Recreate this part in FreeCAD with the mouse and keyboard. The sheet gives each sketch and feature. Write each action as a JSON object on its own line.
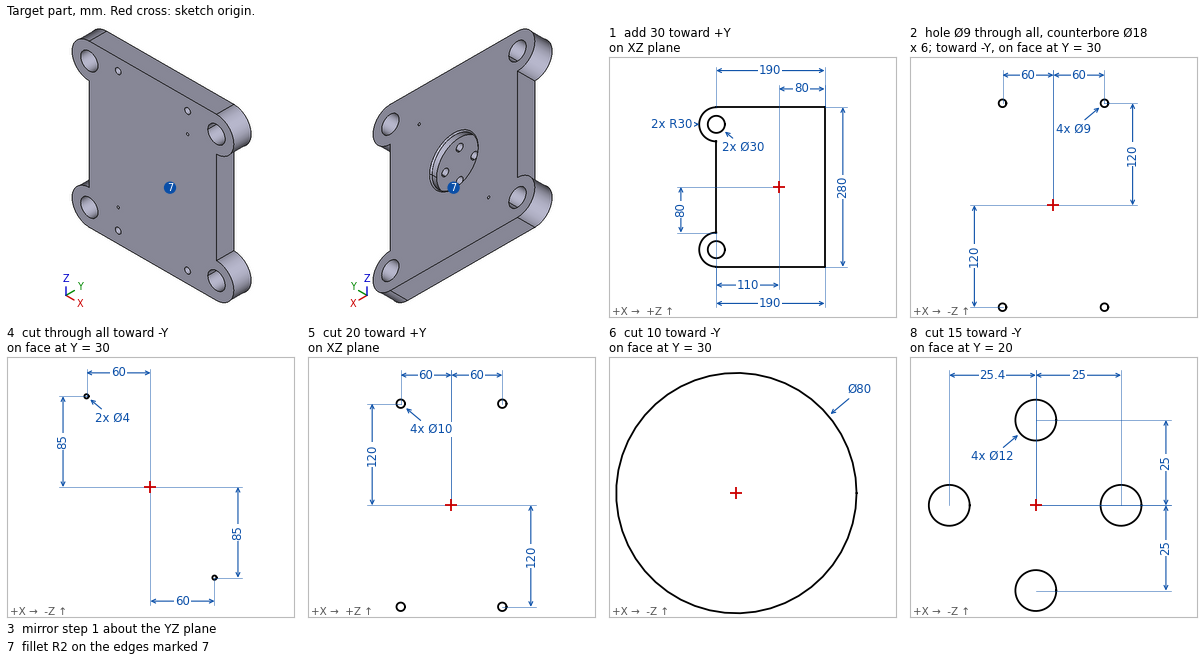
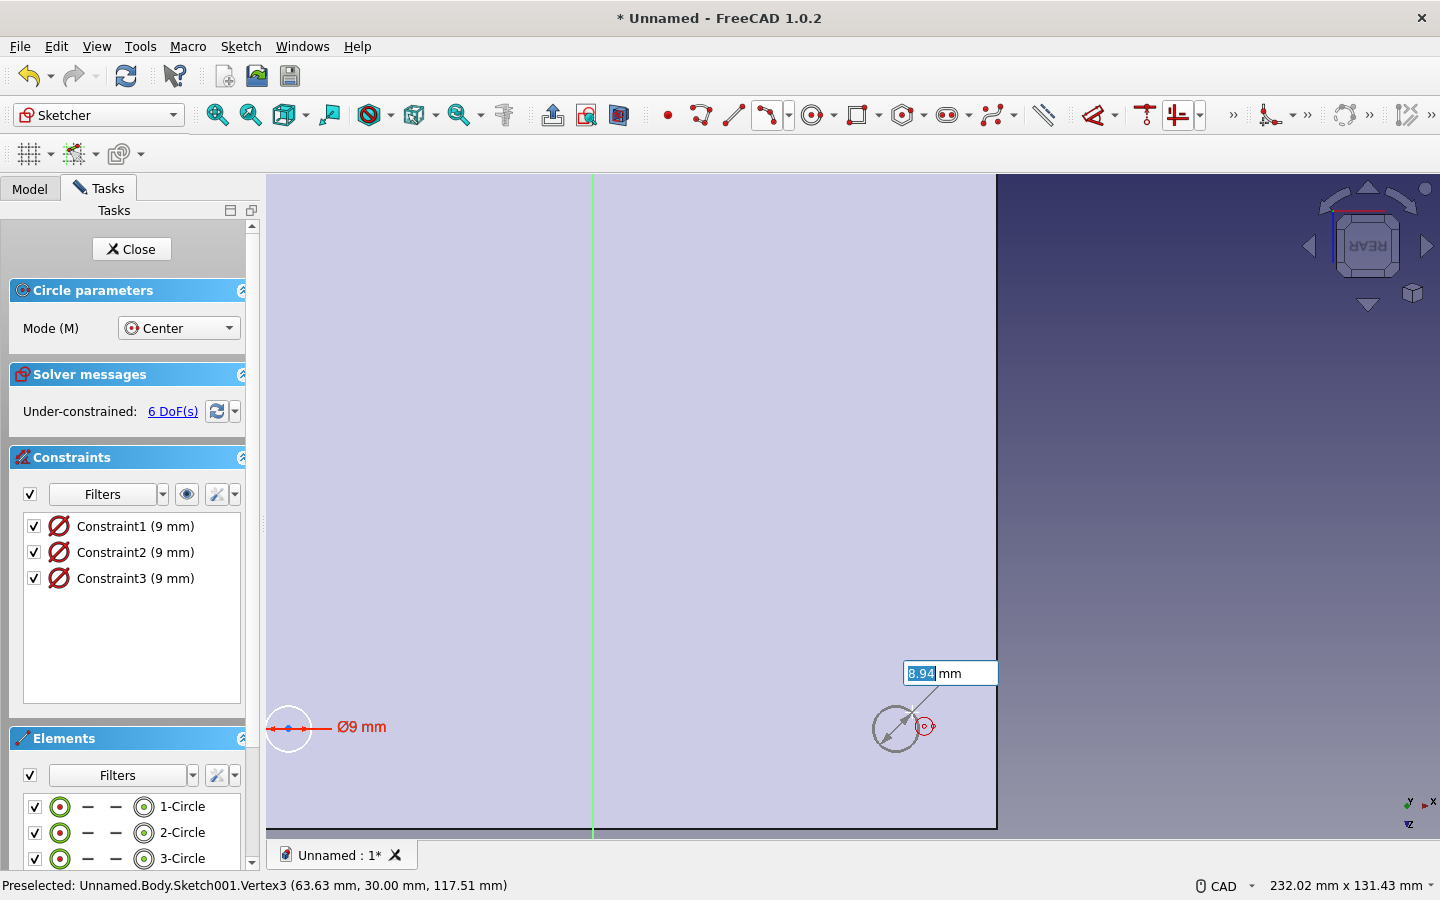
{"action": "type", "text": "9"}
{"action": "key", "text": "Return"}
{"action": "key", "text": "Escape"}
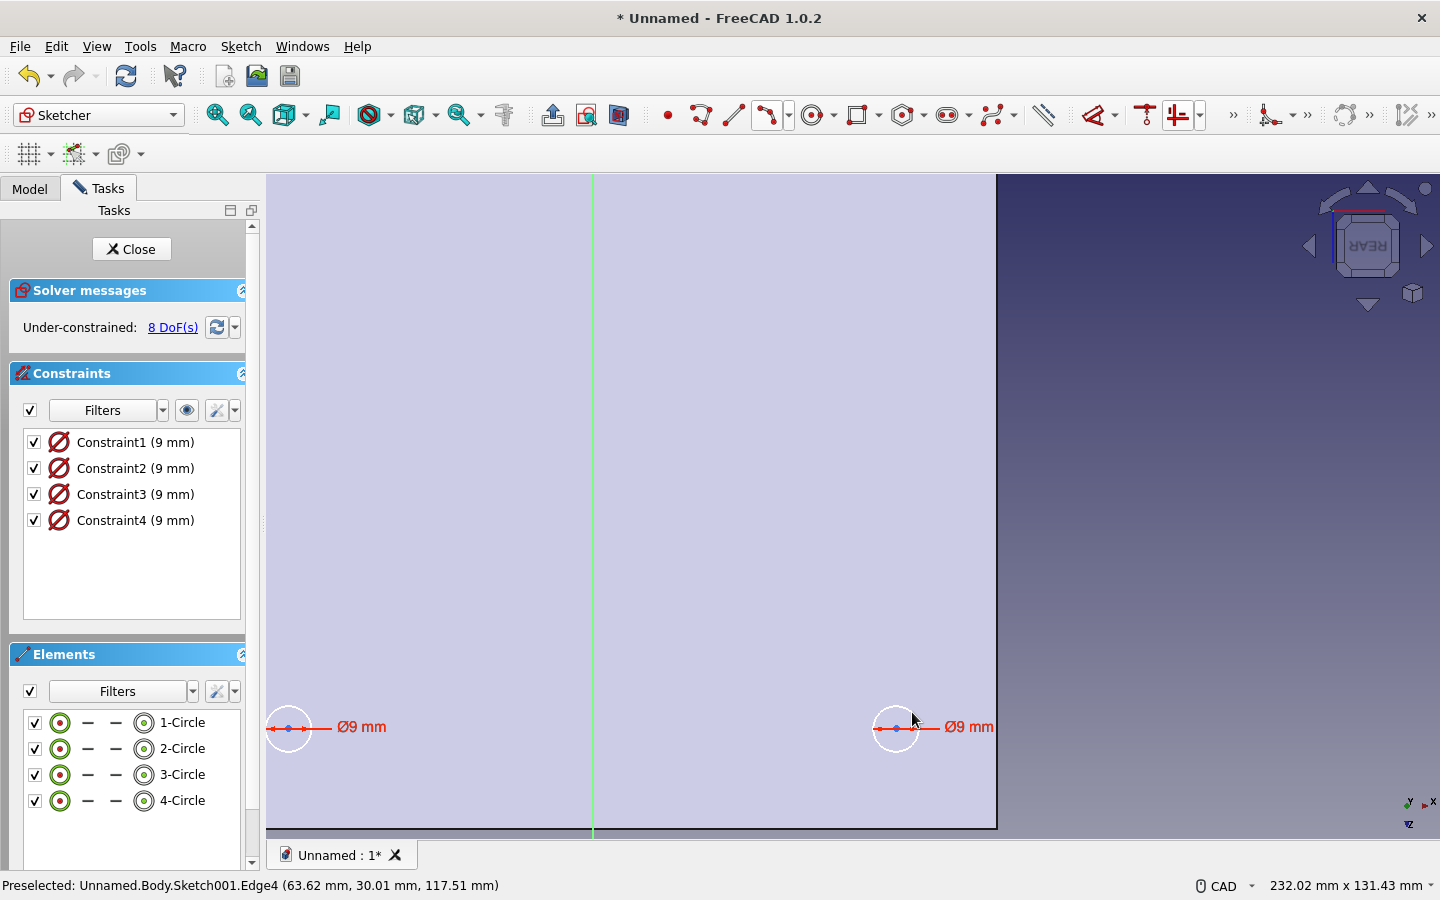
{"action": "scroll", "coordinate": [896, 731], "scroll_direction": "down", "scroll_amount": 5}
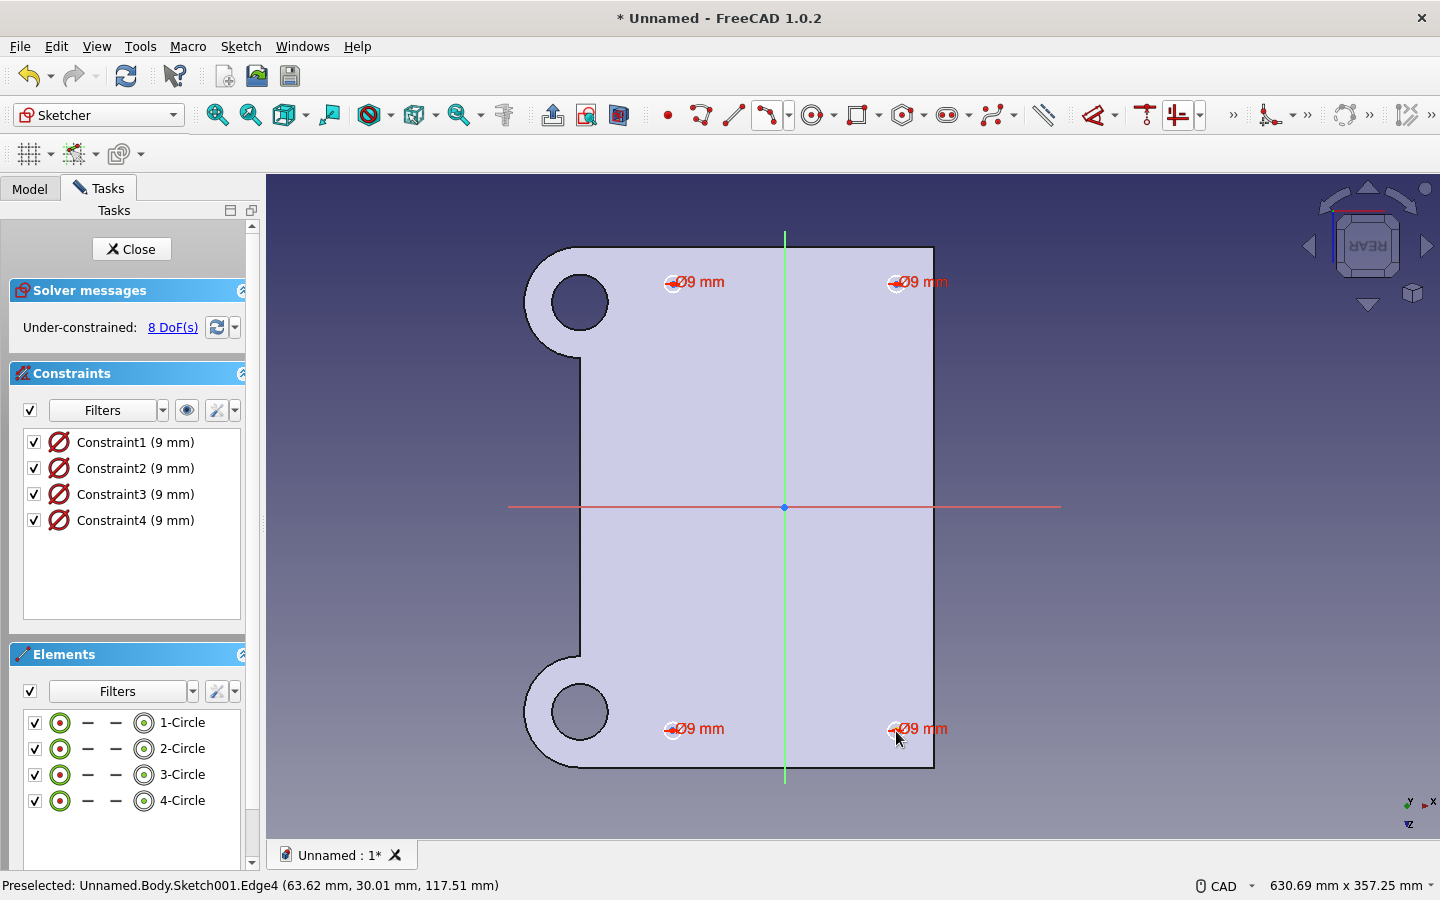
{"action": "left_click", "coordinate": [896, 284]}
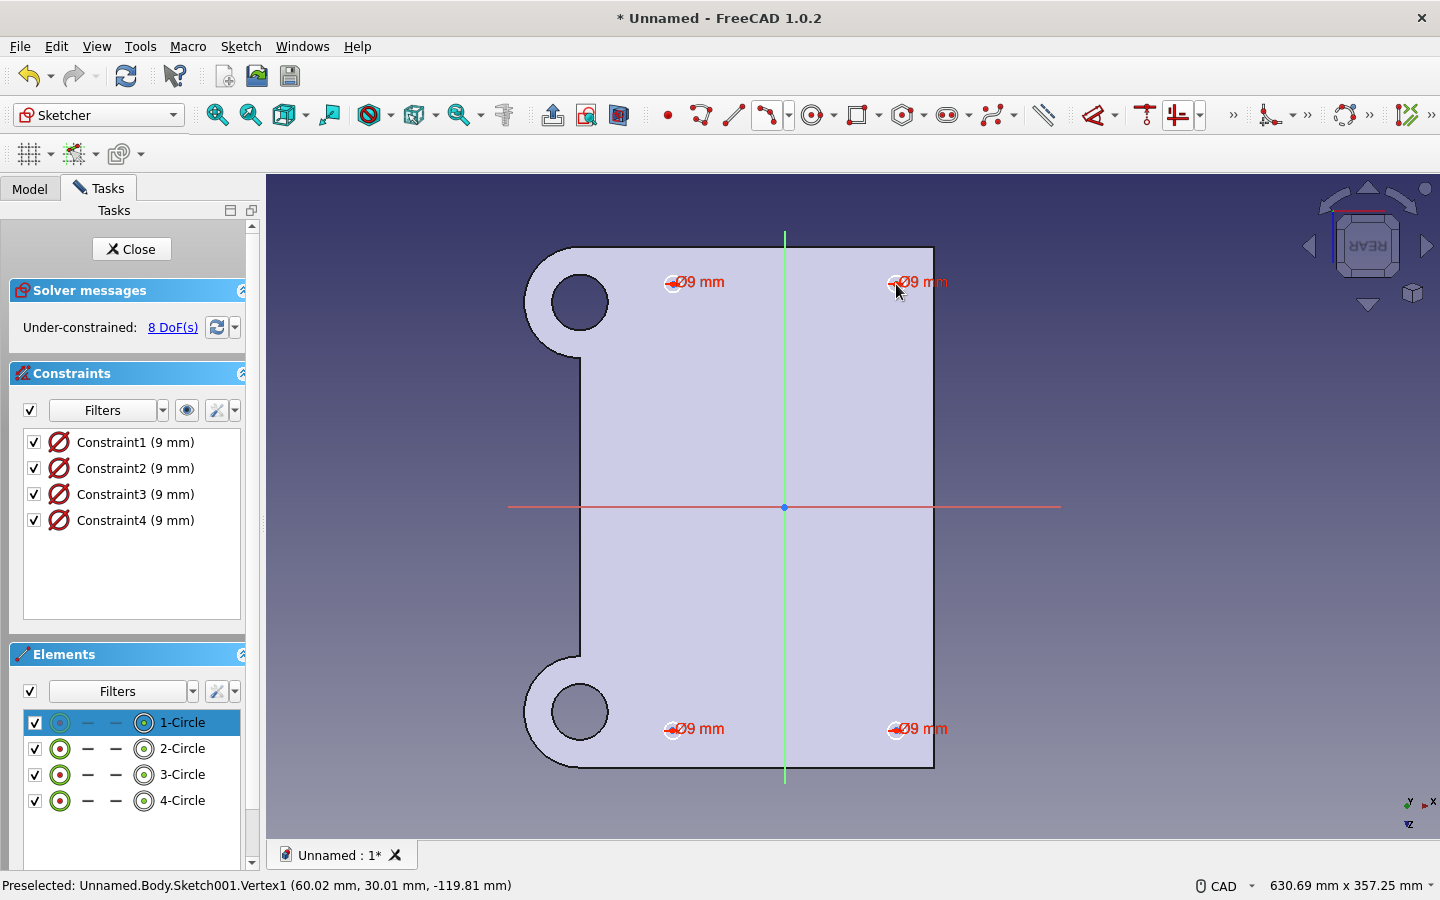
{"action": "left_click", "coordinate": [673, 284]}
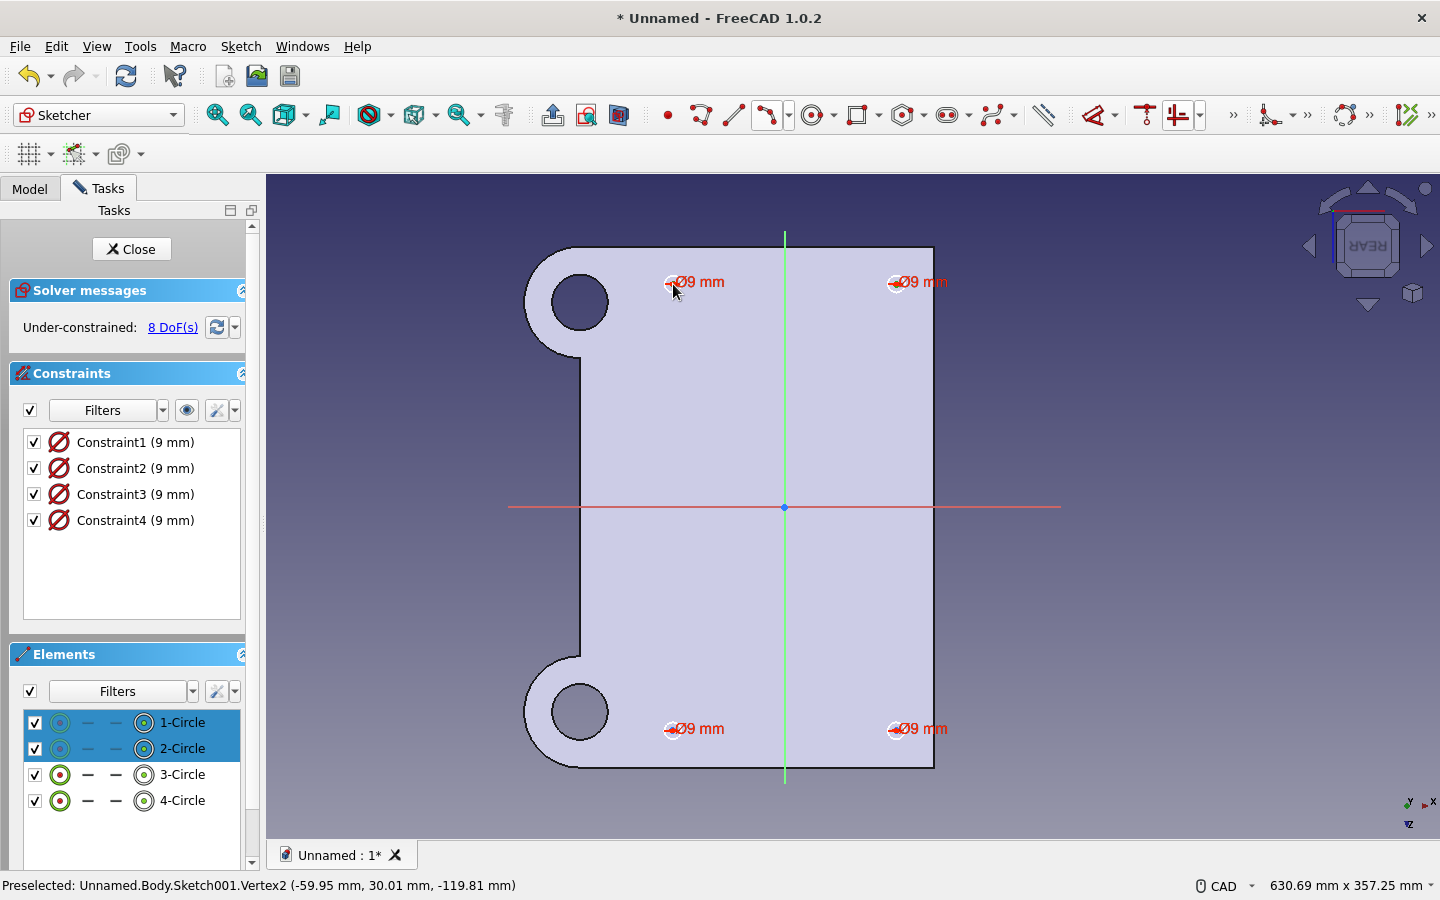
{"action": "key", "text": "h"}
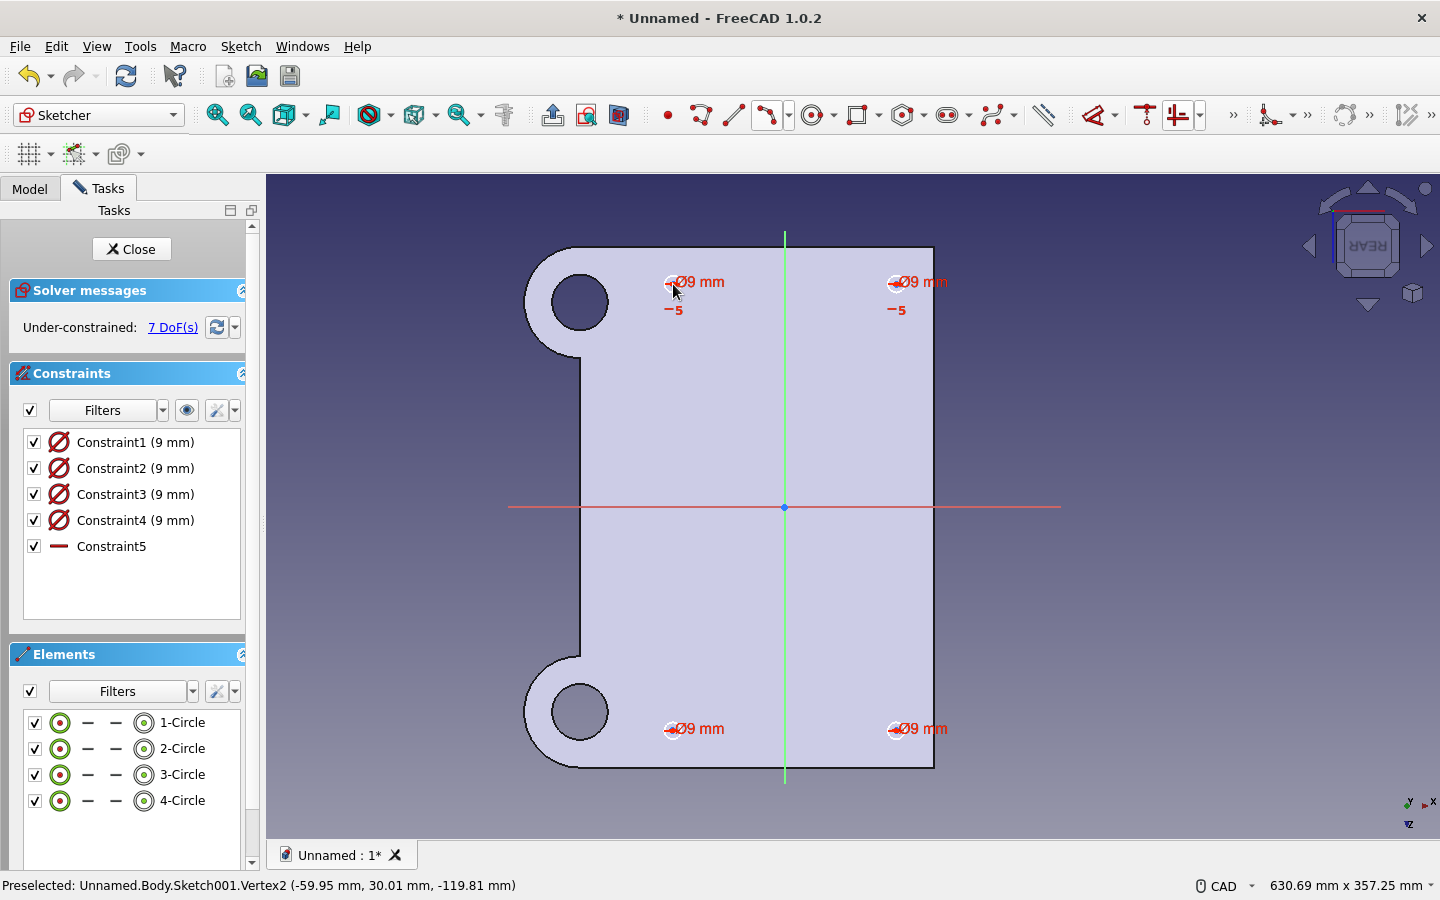
{"action": "left_click", "coordinate": [673, 284]}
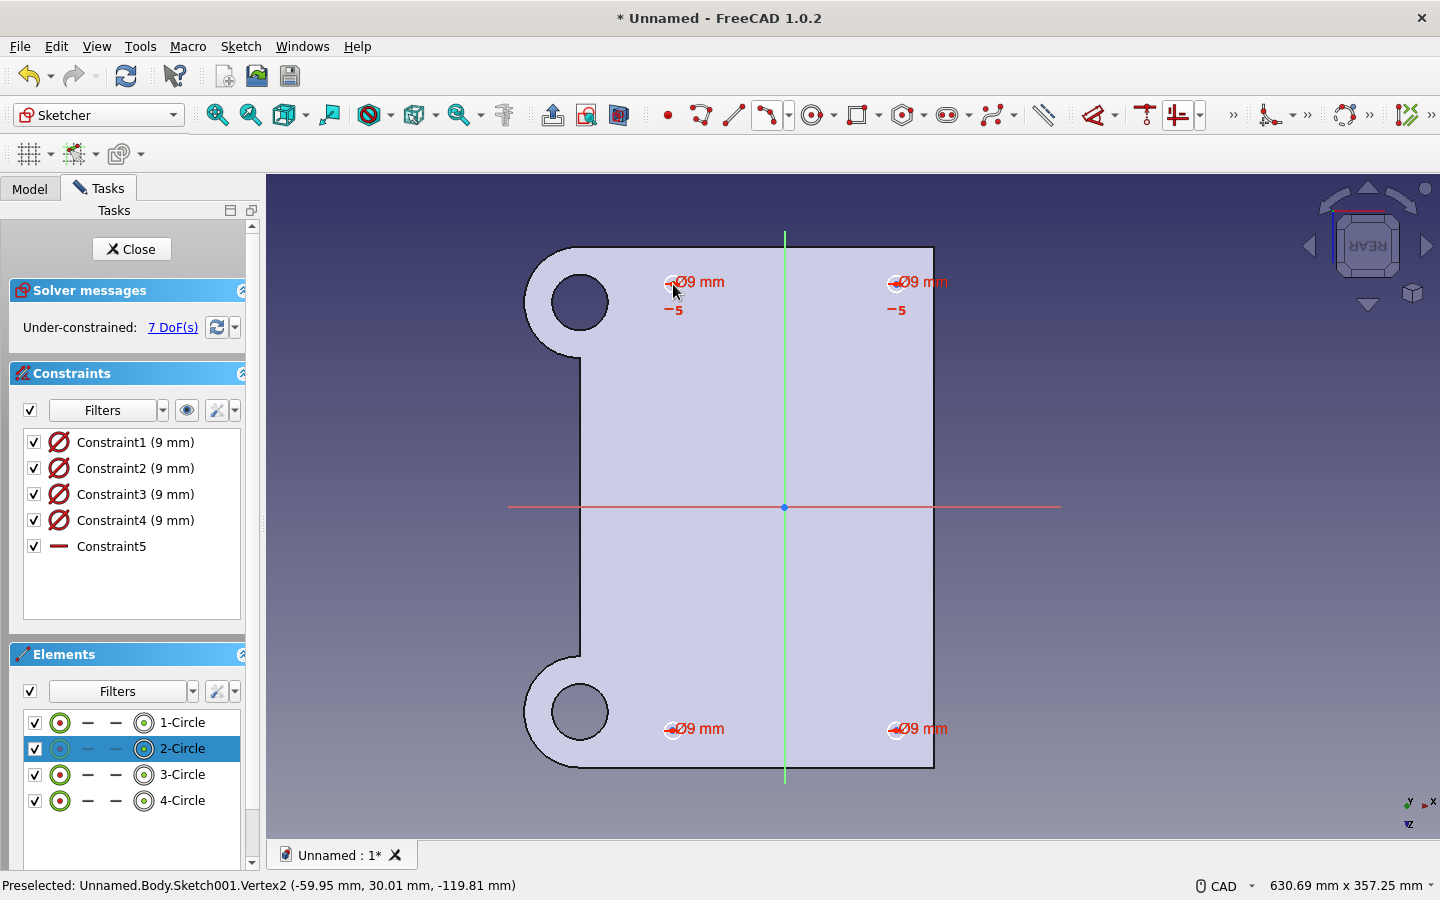
{"action": "left_click", "coordinate": [673, 731]}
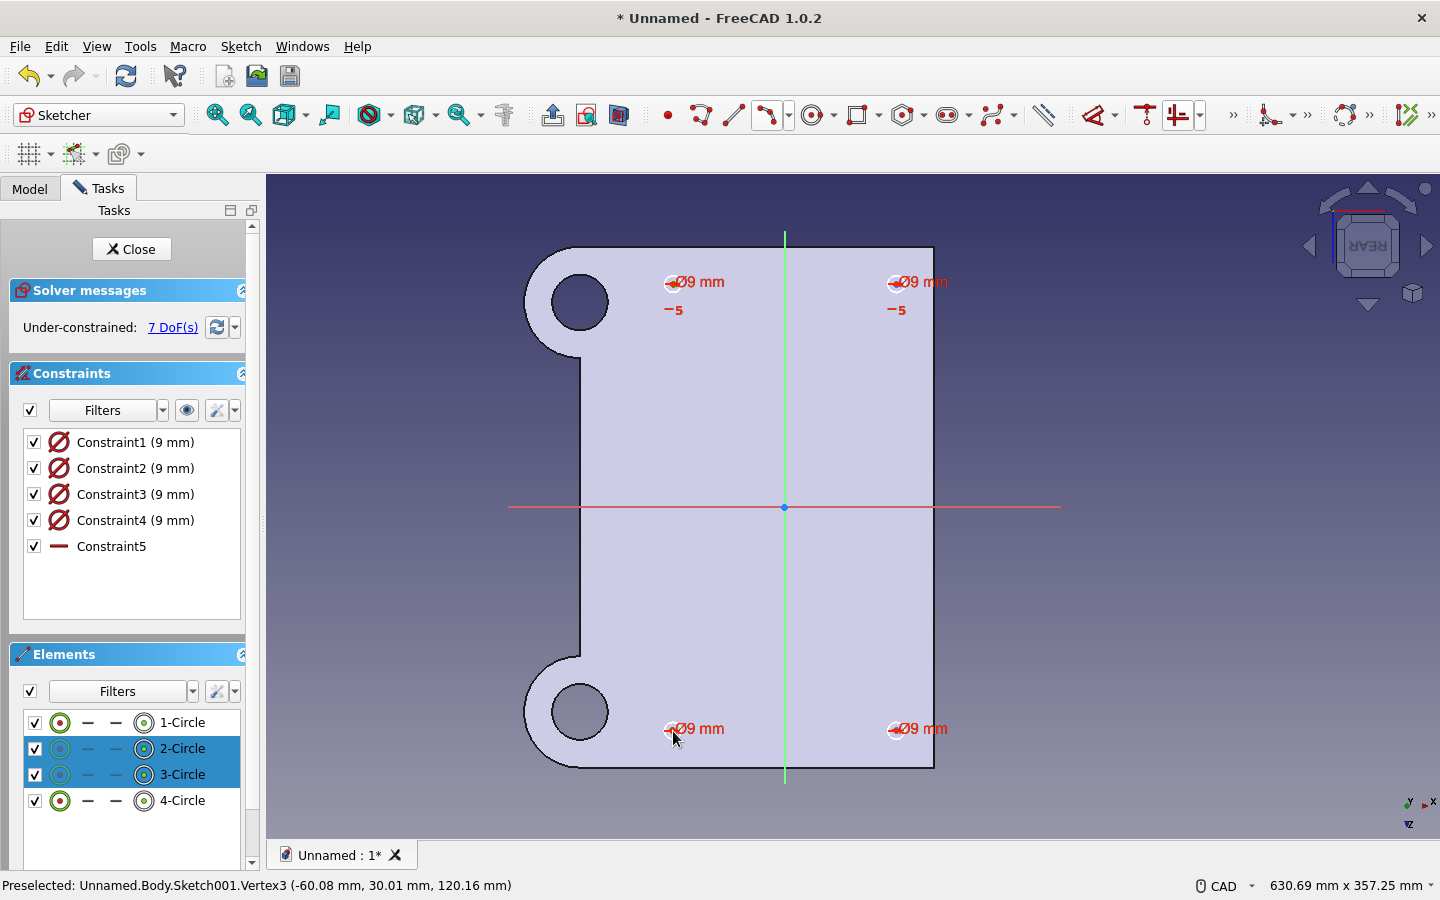
{"action": "key", "text": "v"}